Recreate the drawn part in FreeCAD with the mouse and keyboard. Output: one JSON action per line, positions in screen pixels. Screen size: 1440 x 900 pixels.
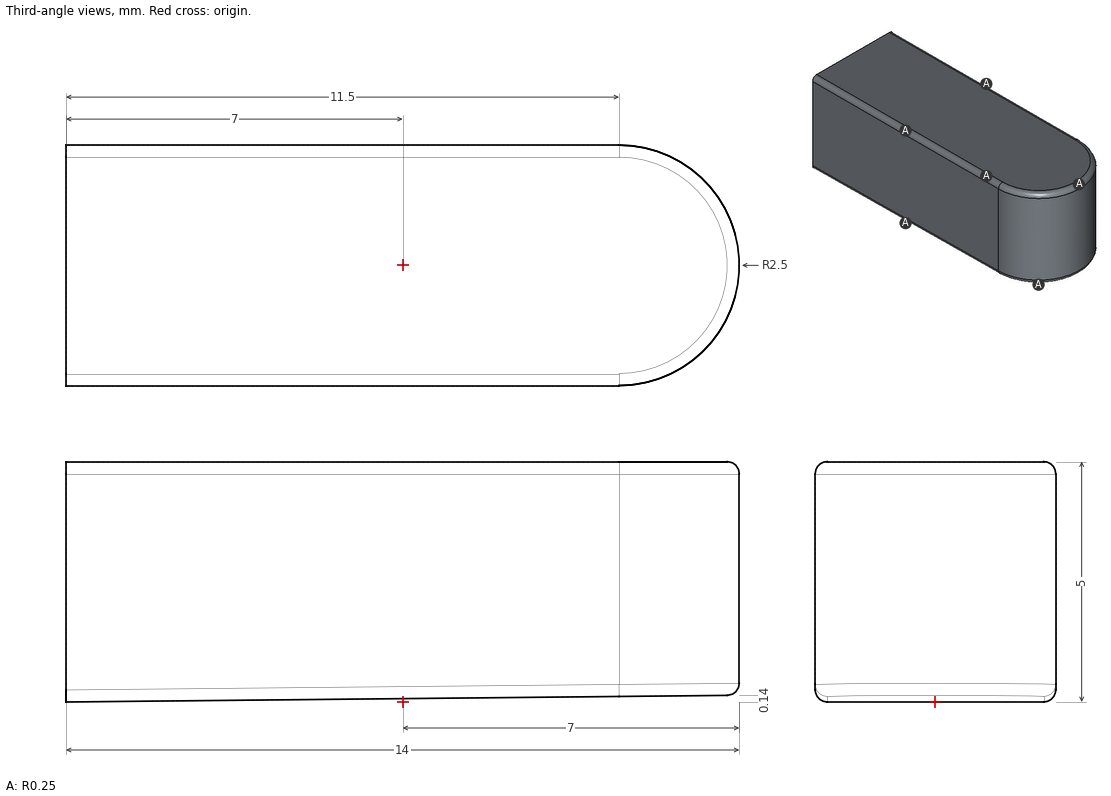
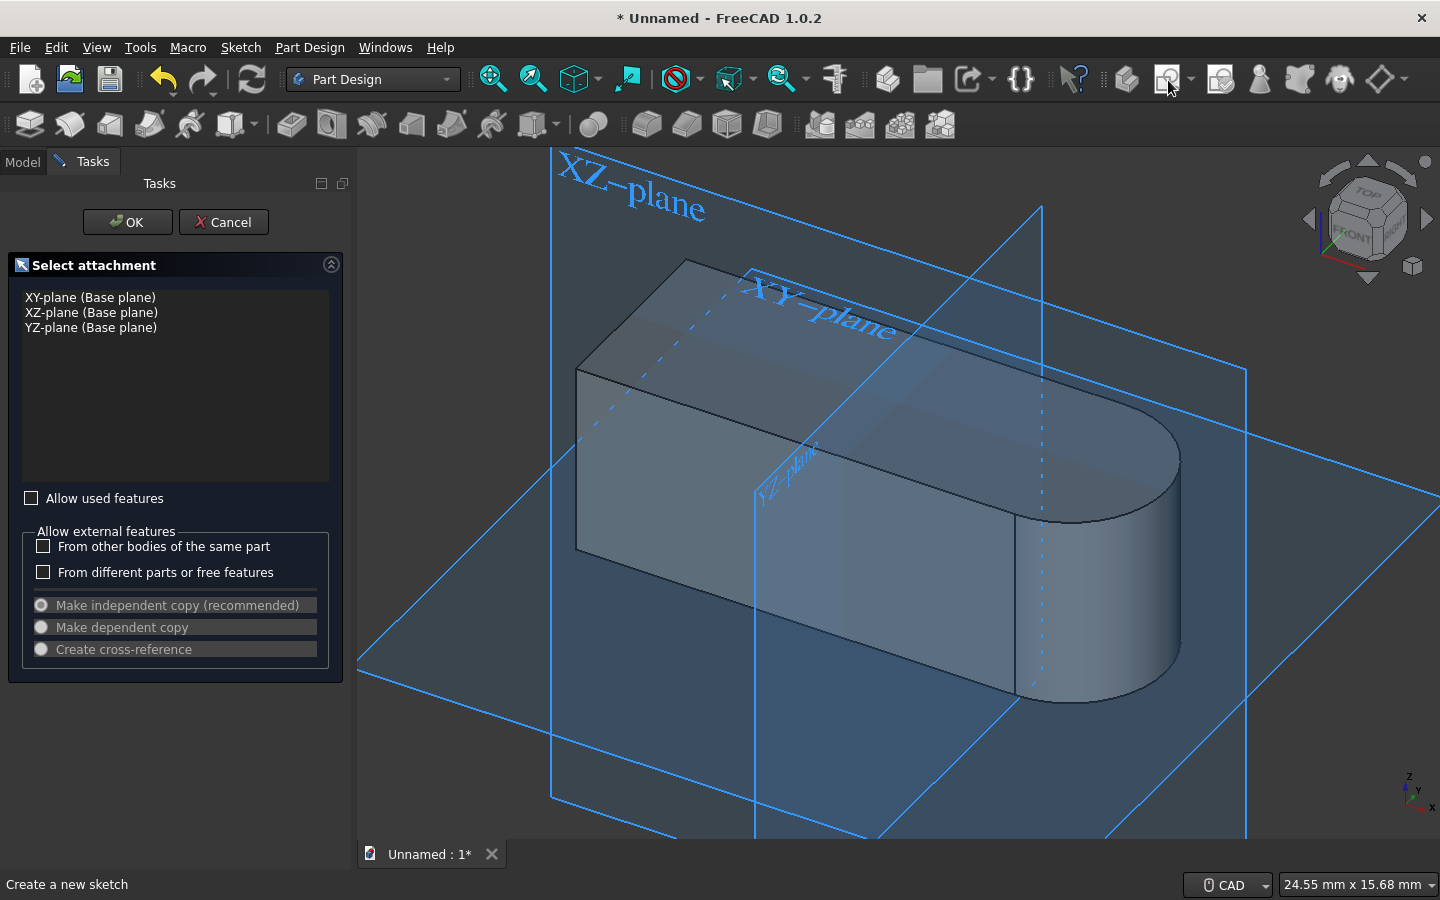
{"action": "left_click", "coordinate": [82, 312]}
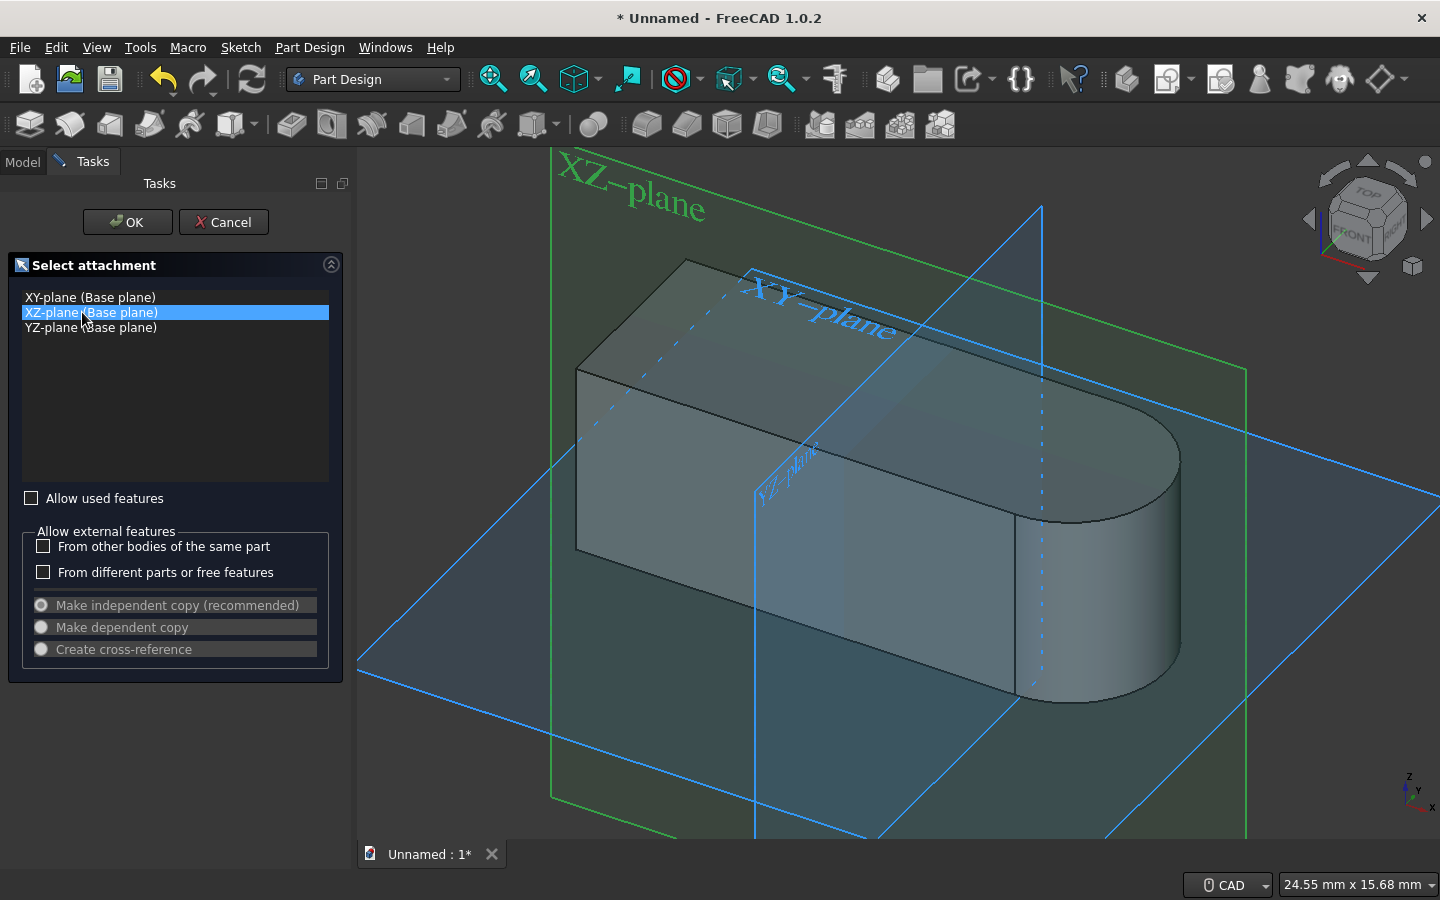
{"action": "left_click", "coordinate": [128, 222]}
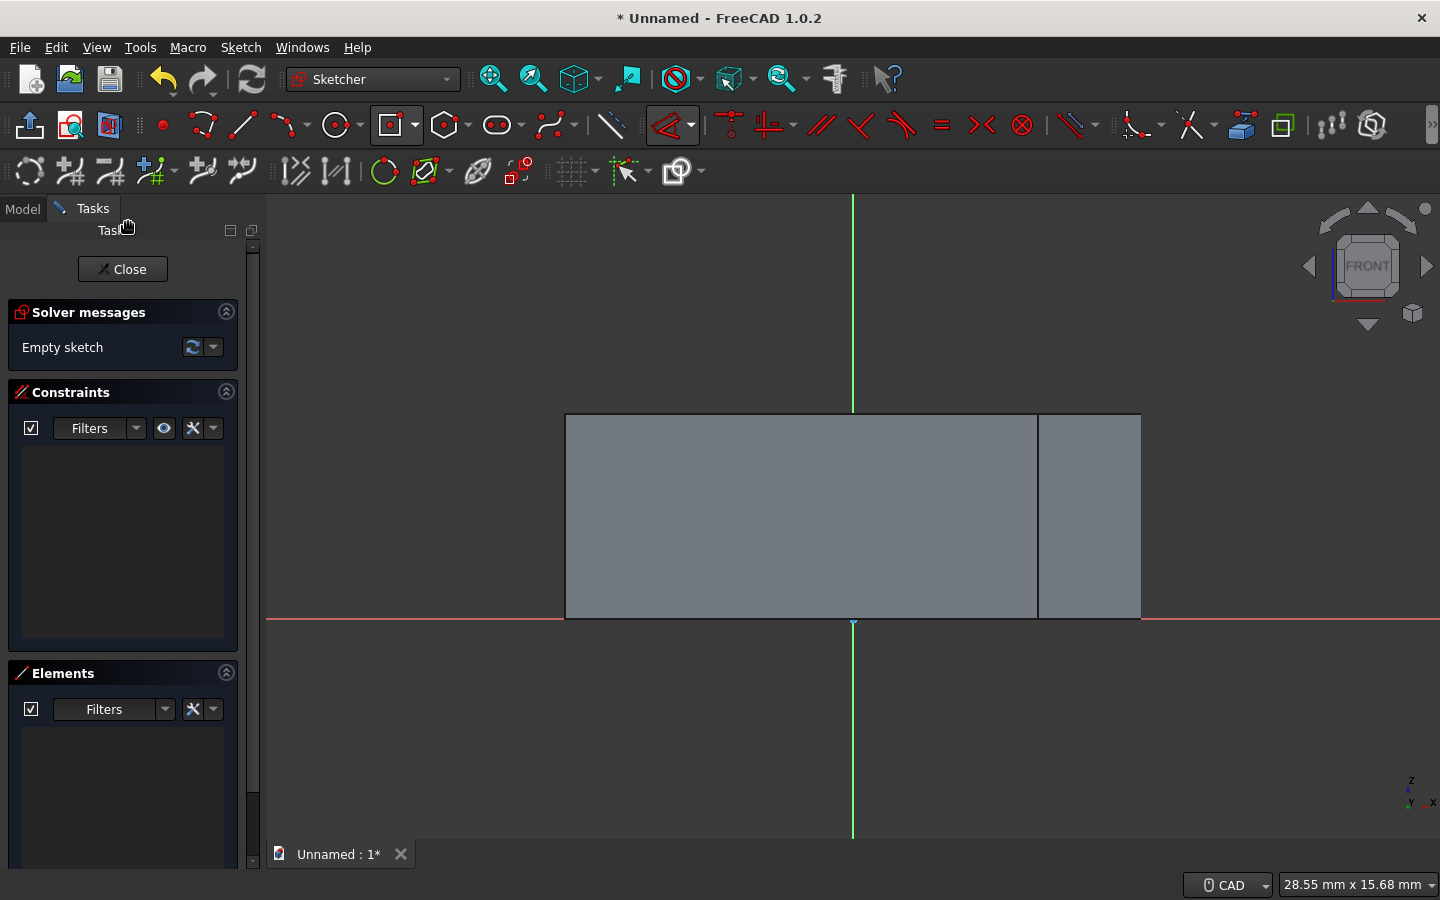
{"action": "left_click", "coordinate": [110, 126]}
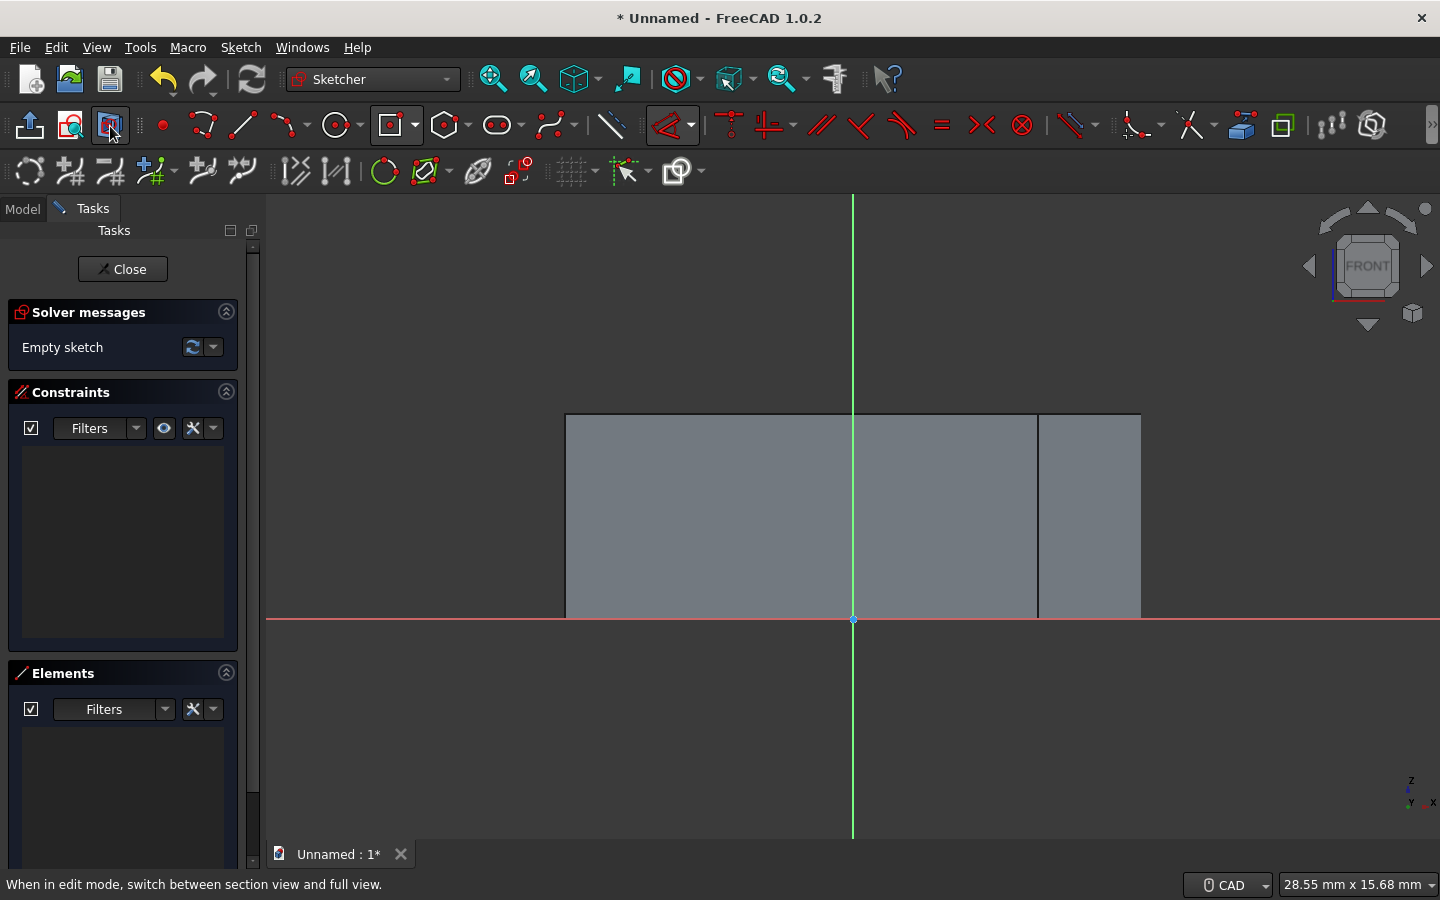
{"action": "left_click", "coordinate": [204, 126]}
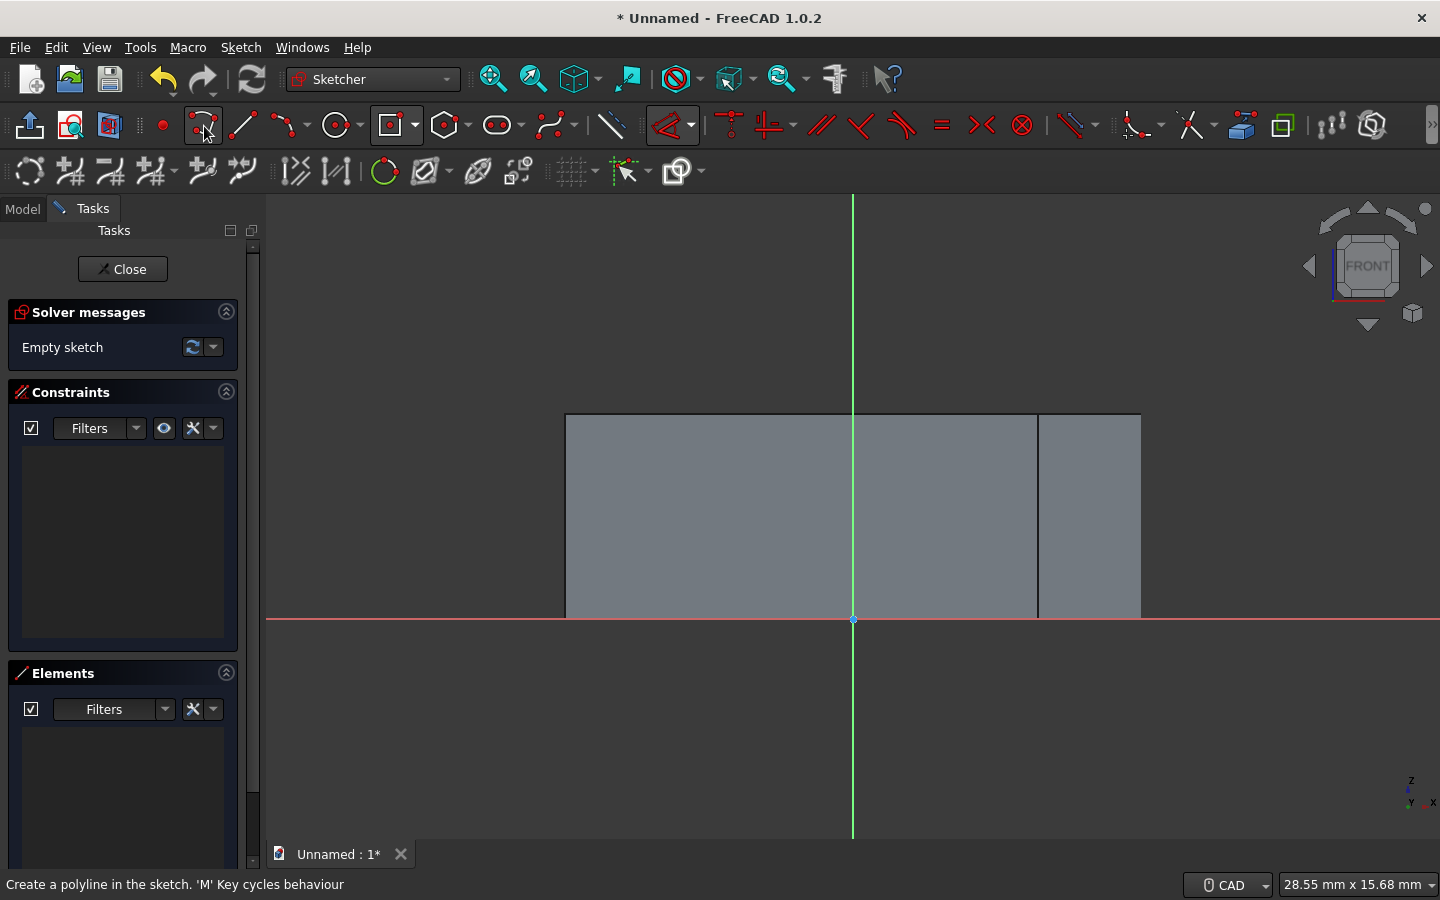
{"action": "left_click", "coordinate": [1141, 619]}
{"action": "left_click", "coordinate": [565, 610]}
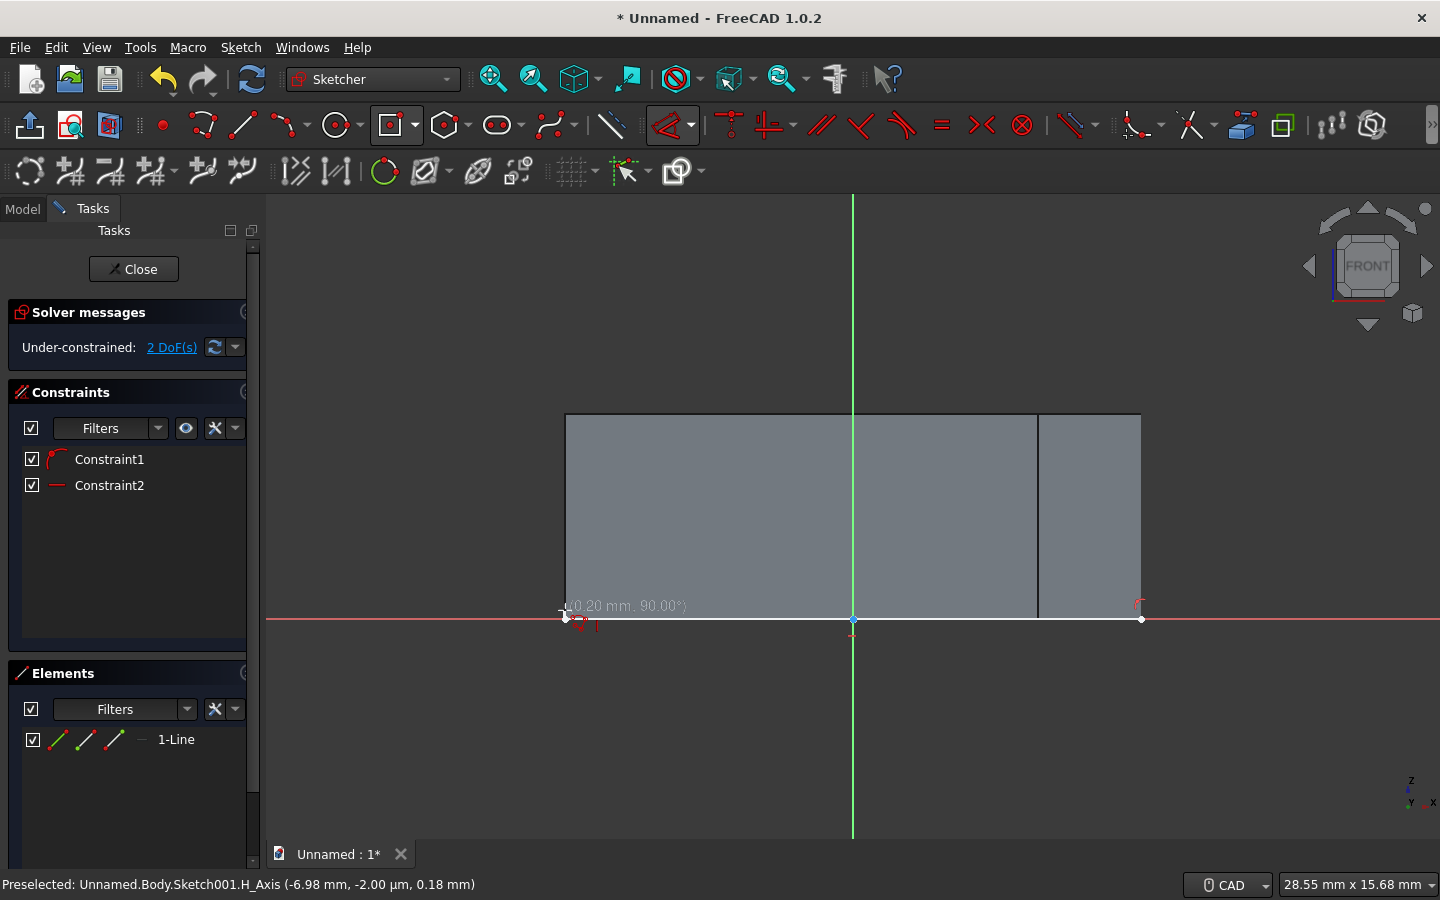
{"action": "scroll", "coordinate": [1141, 614], "scroll_direction": "up", "scroll_amount": 6}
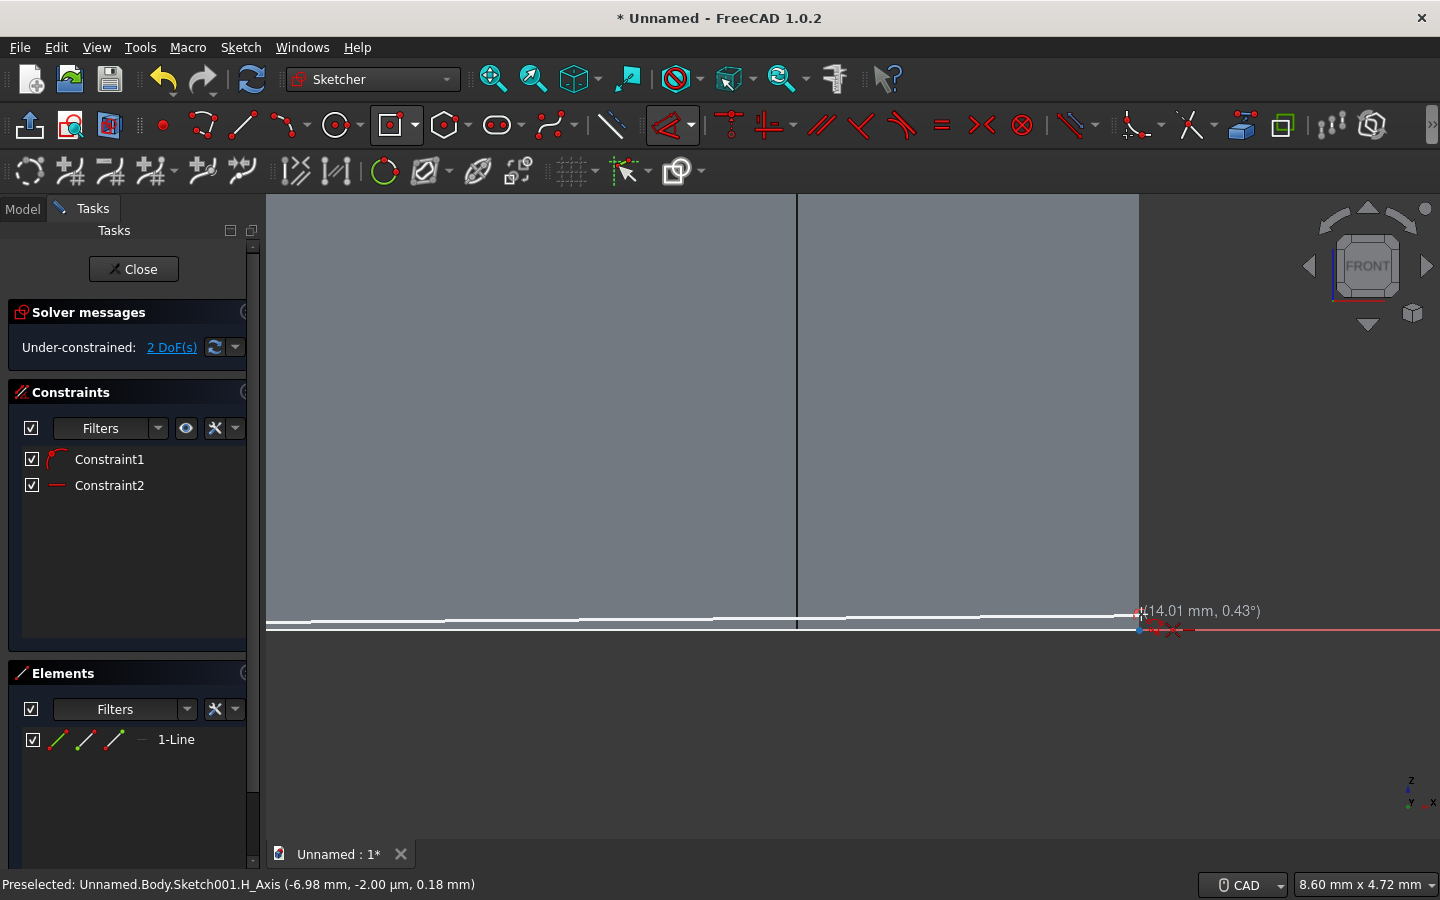
{"action": "left_click", "coordinate": [1139, 512]}
{"action": "left_click", "coordinate": [1139, 630]}
{"action": "key", "text": "Escape"}
{"action": "key", "text": "Escape"}